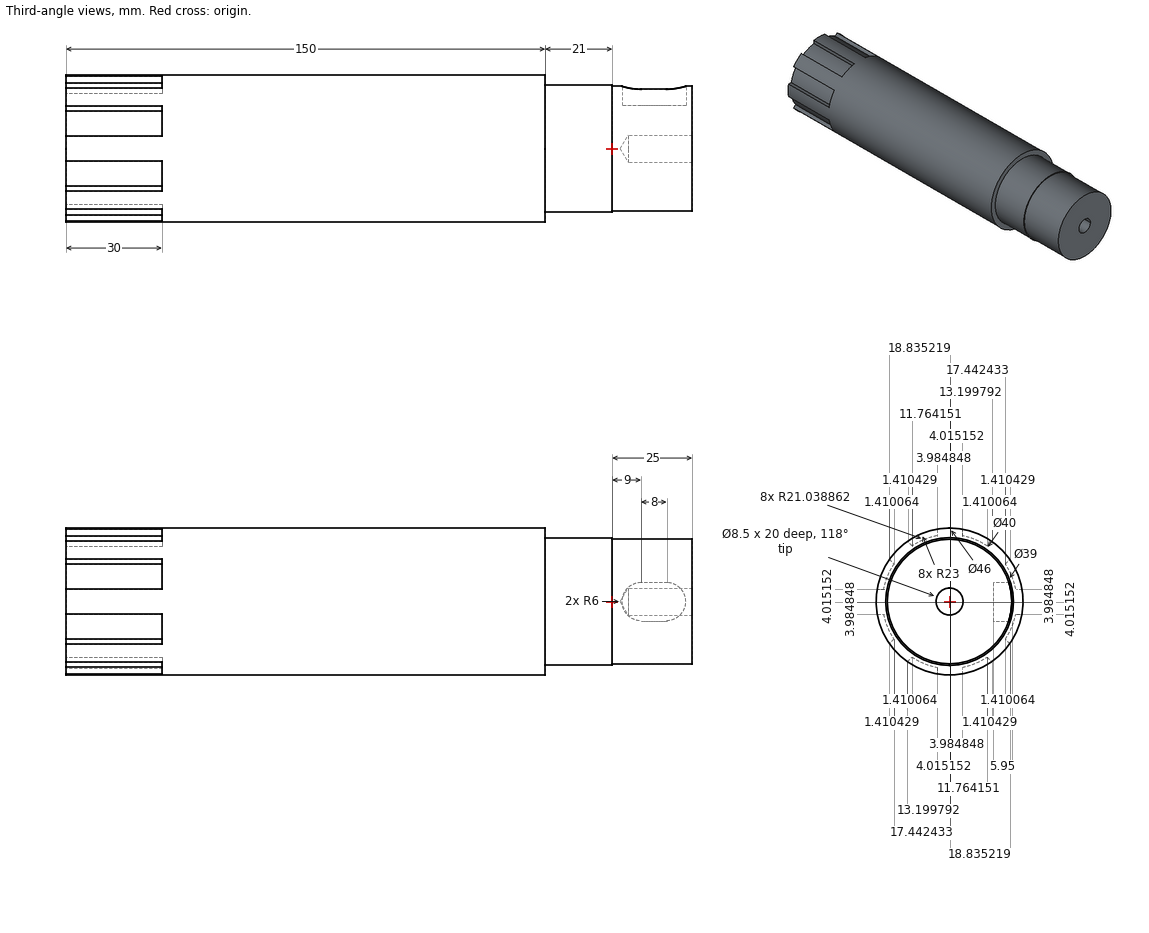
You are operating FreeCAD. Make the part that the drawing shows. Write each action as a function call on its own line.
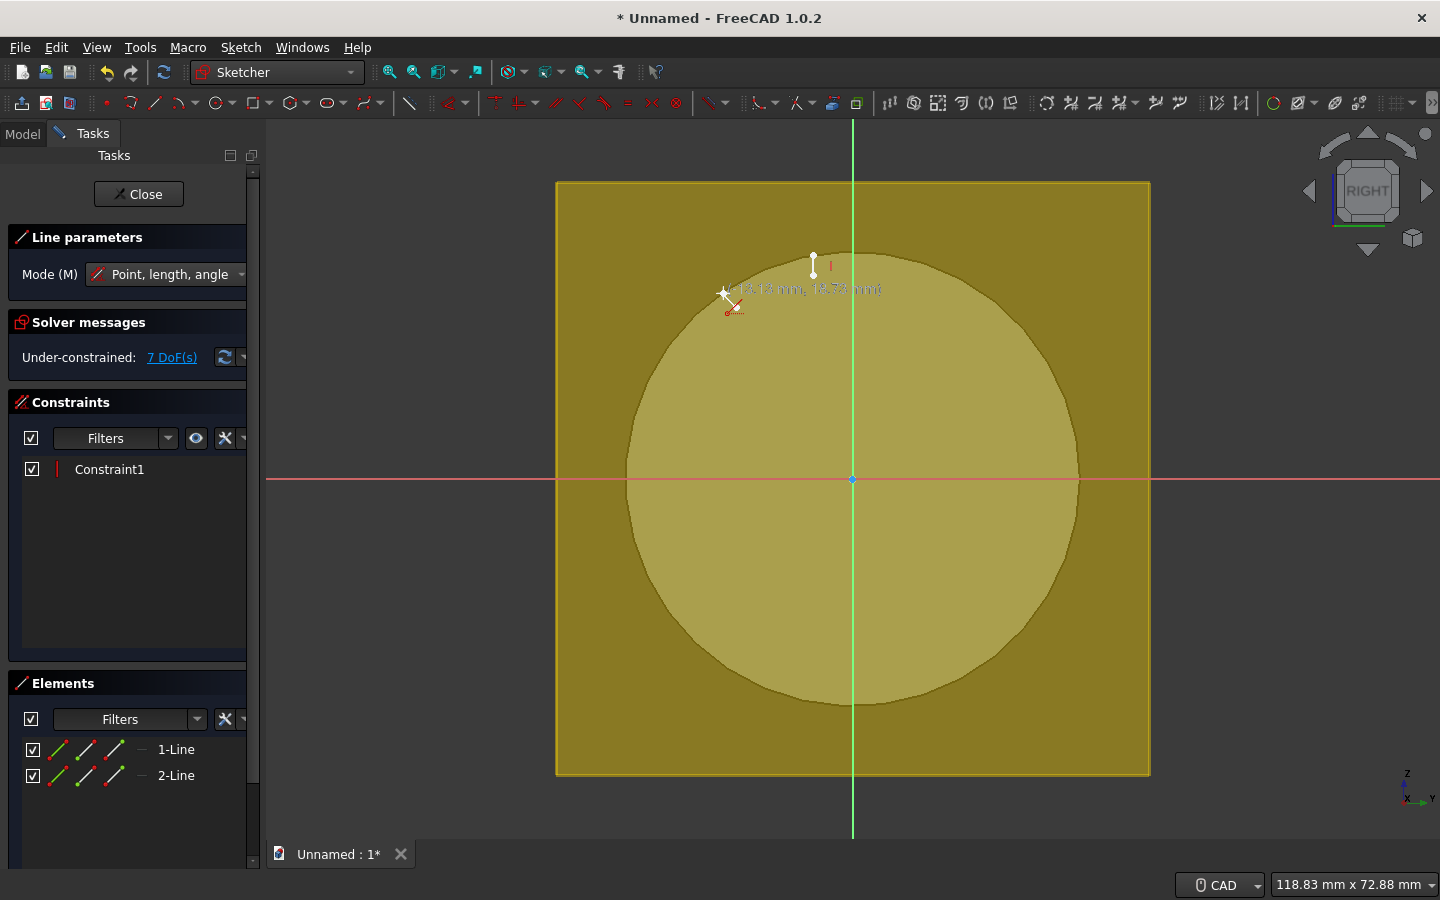
key(g)
key(3)
key(a)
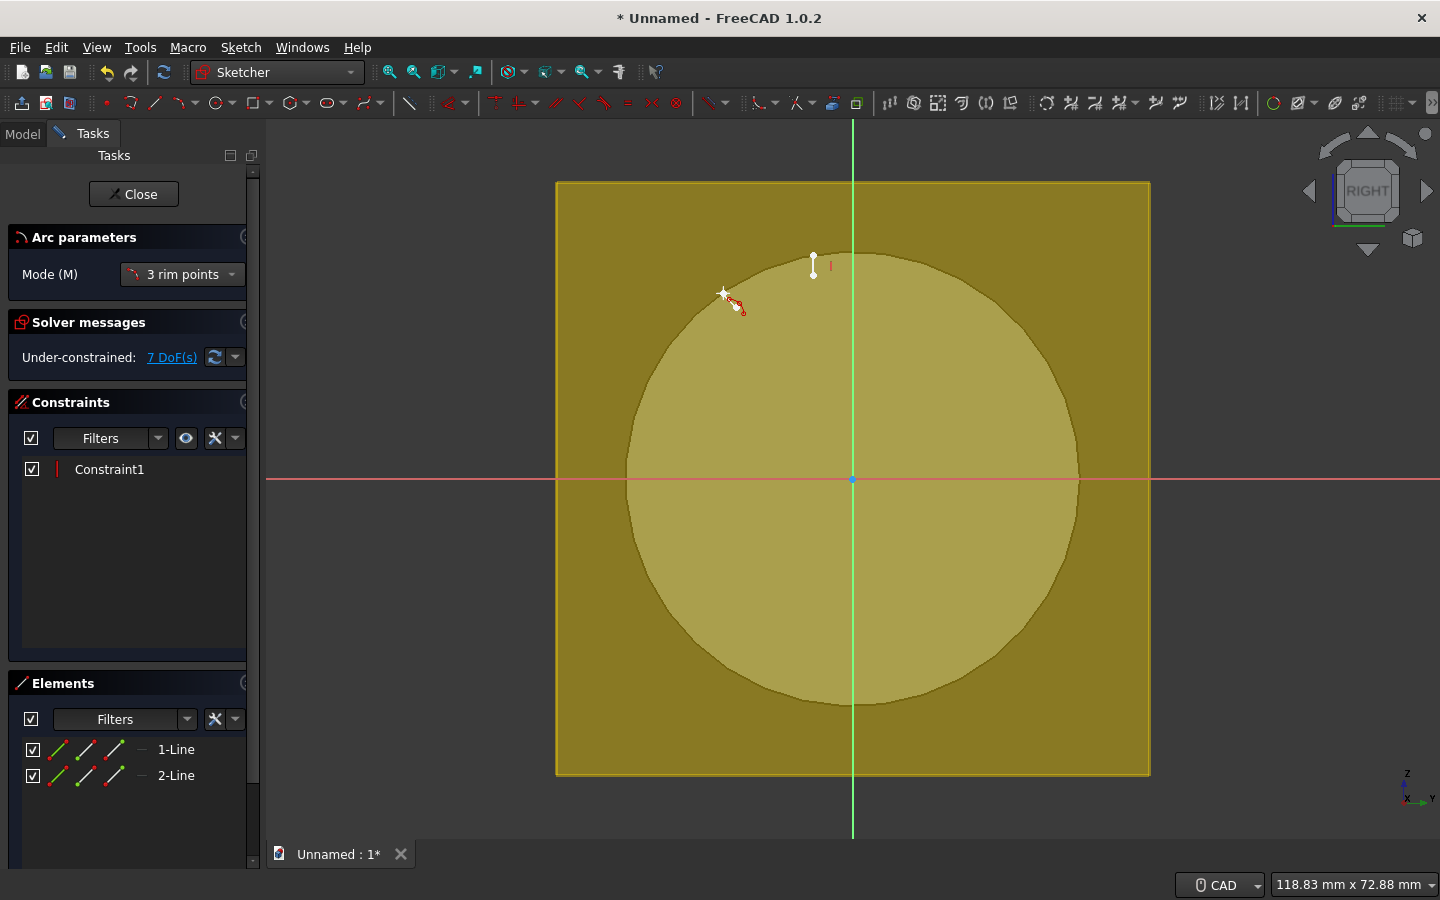
scroll(813, 275, up, 3)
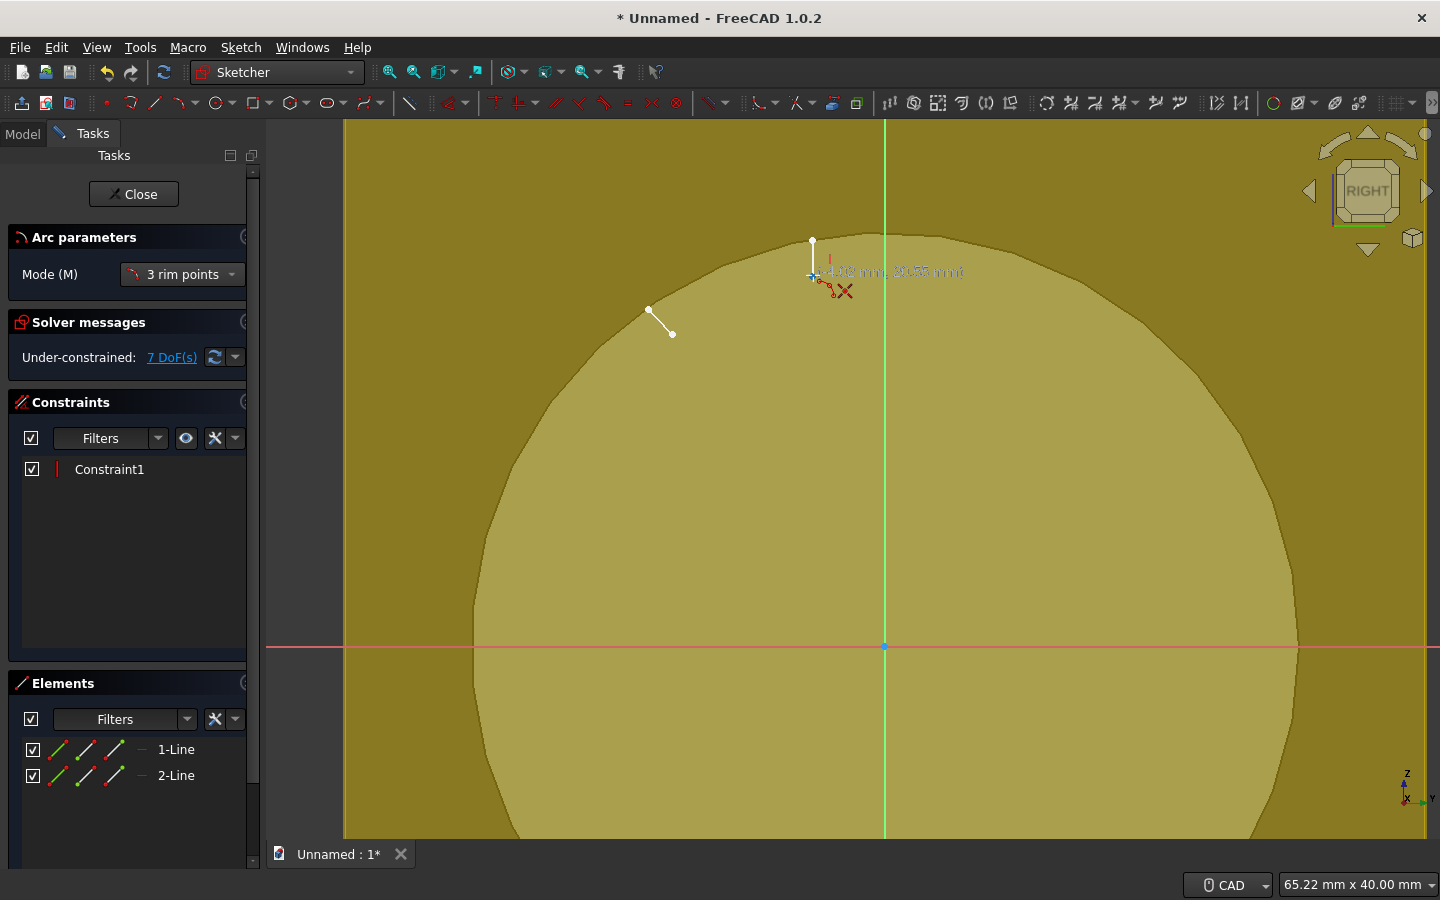
click(813, 277)
click(672, 335)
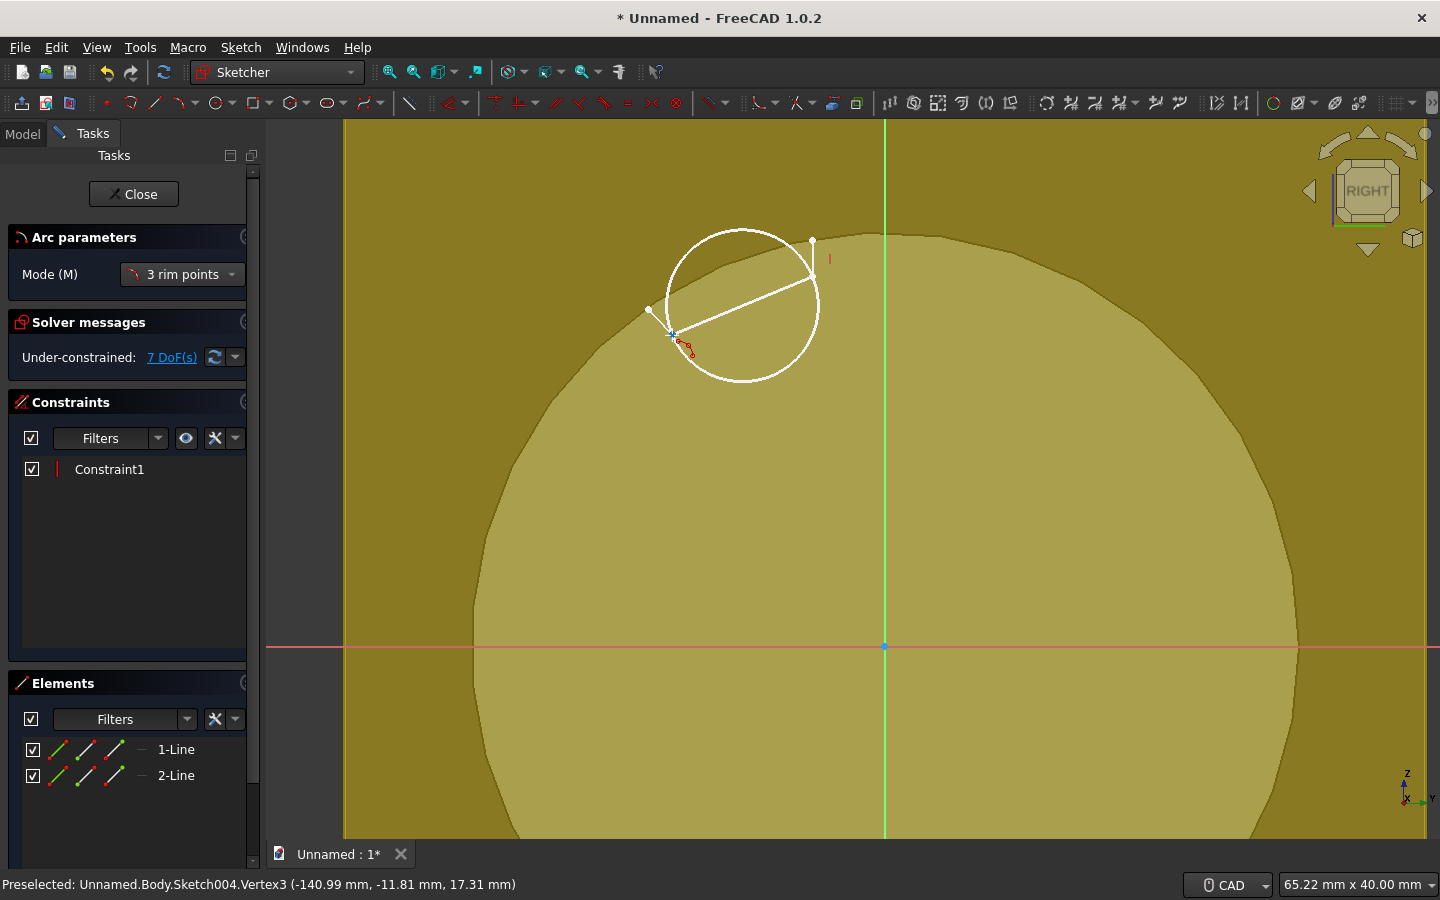
scroll(740, 297, up, 4)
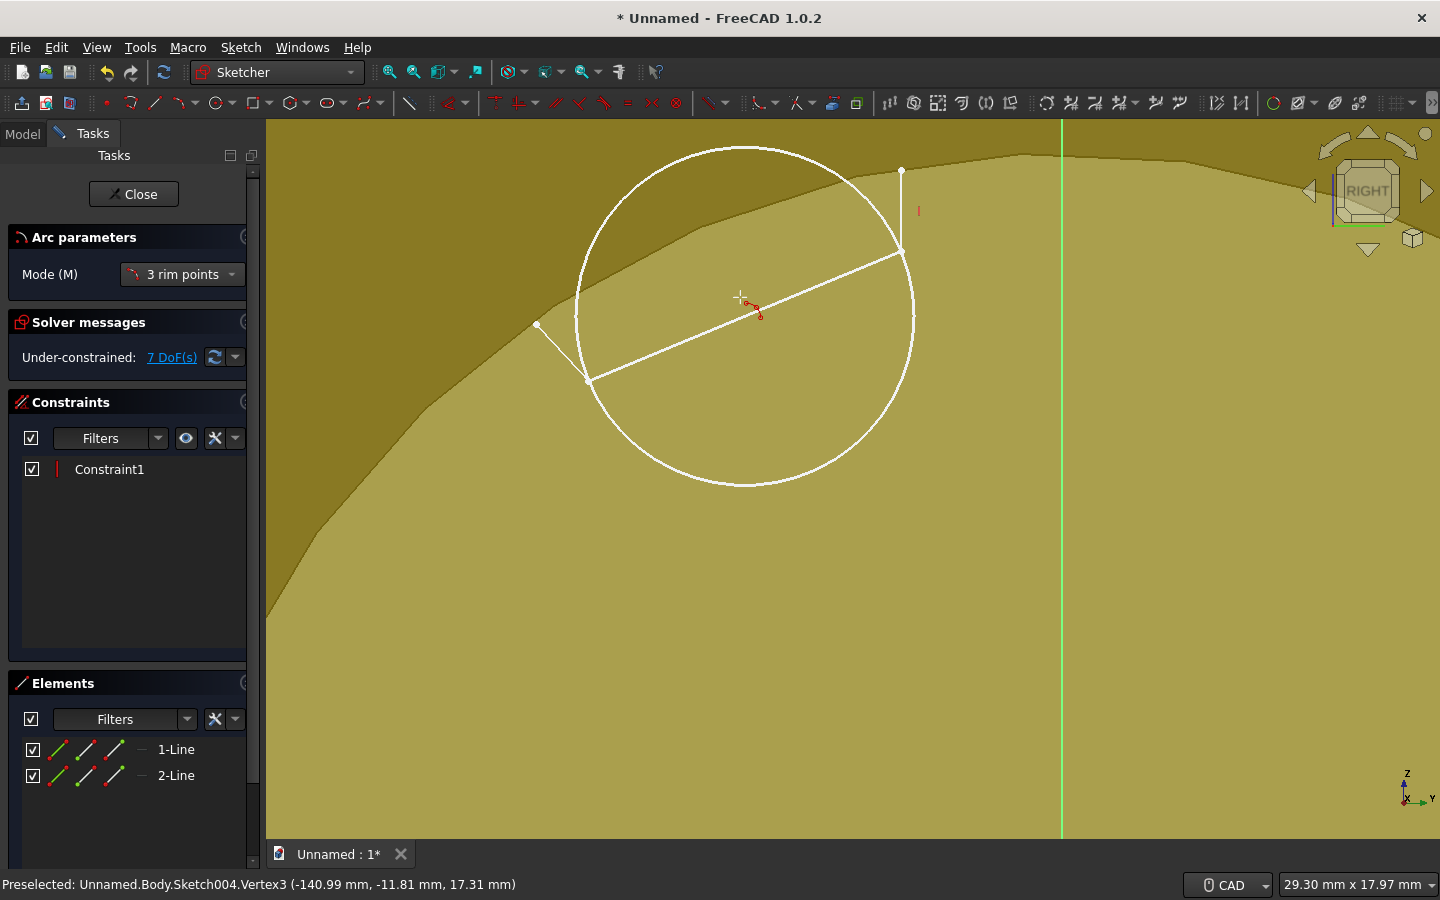
click(740, 296)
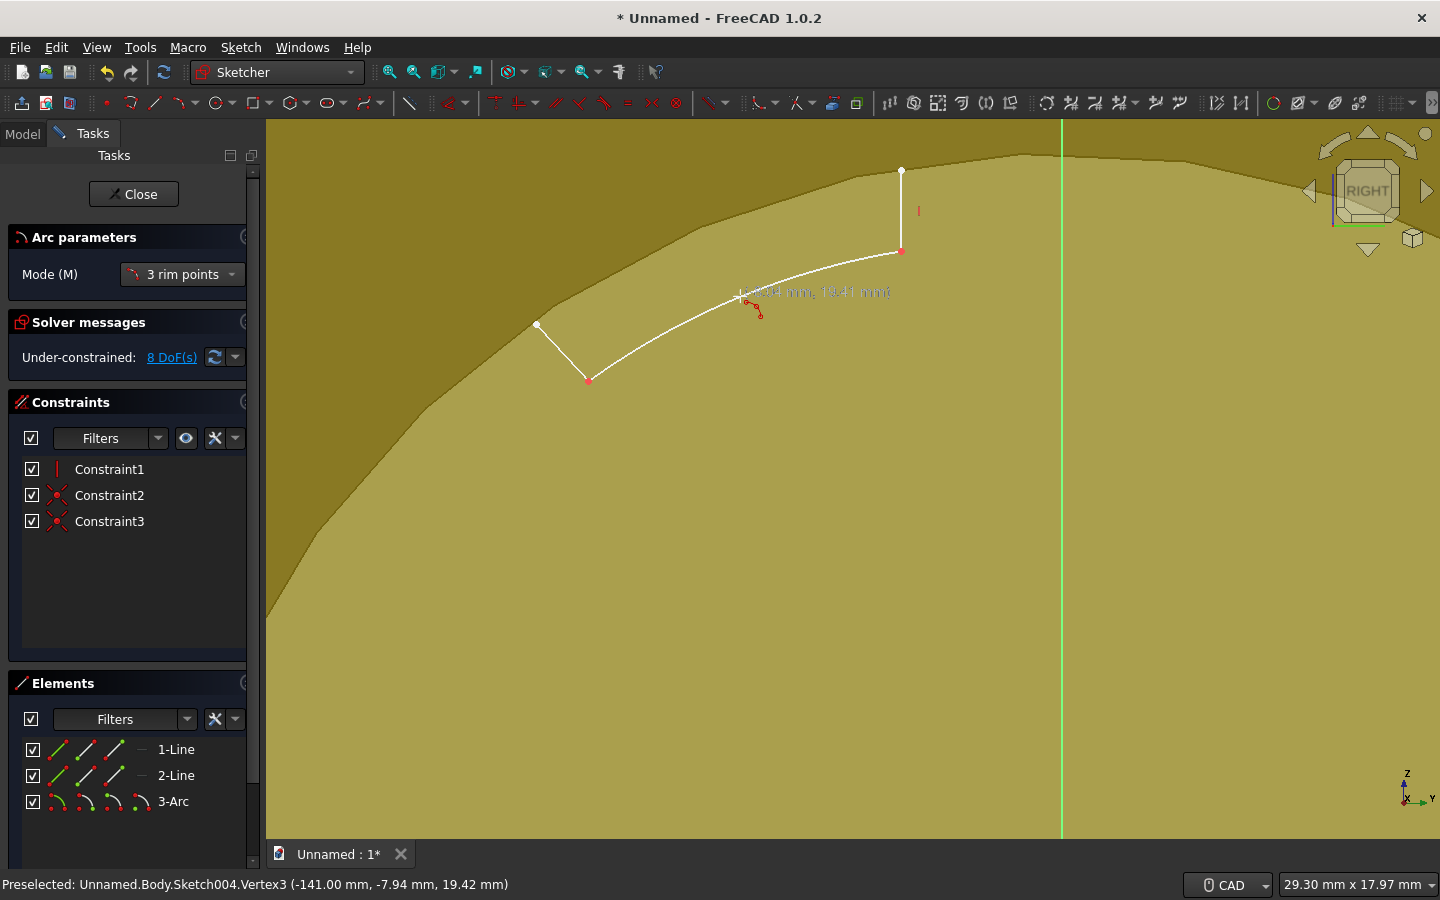
click(536, 324)
click(901, 170)
click(710, 223)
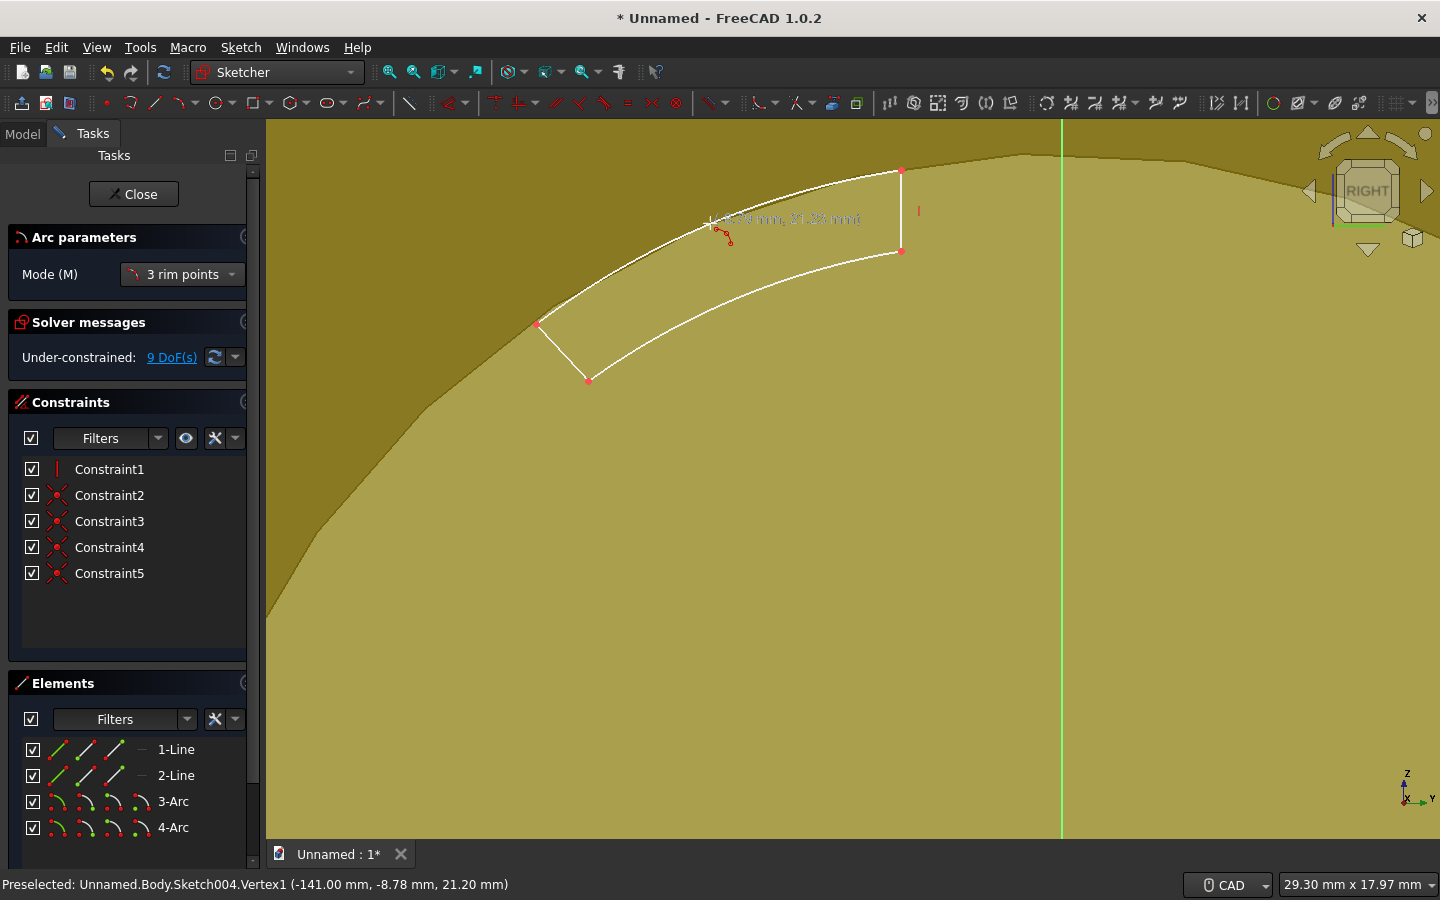
click(156, 104)